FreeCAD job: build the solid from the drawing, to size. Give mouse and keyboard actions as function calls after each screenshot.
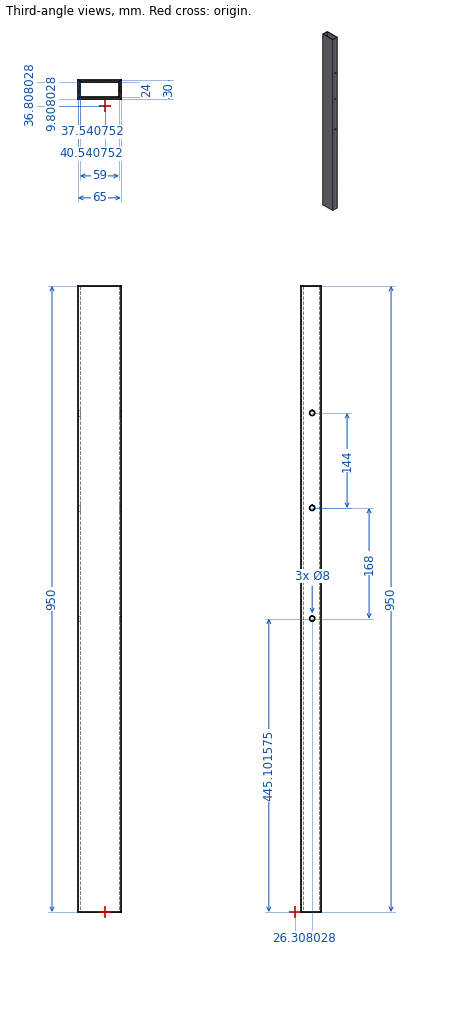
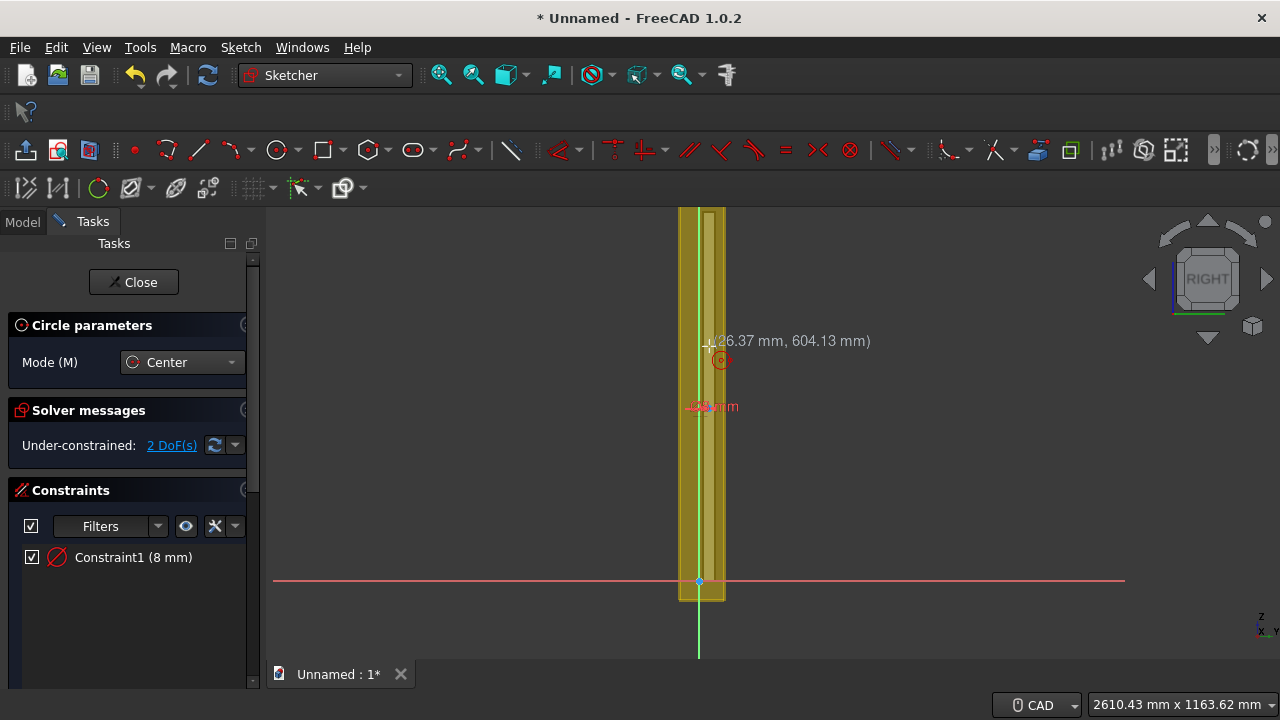
scroll(709, 343, up, 3)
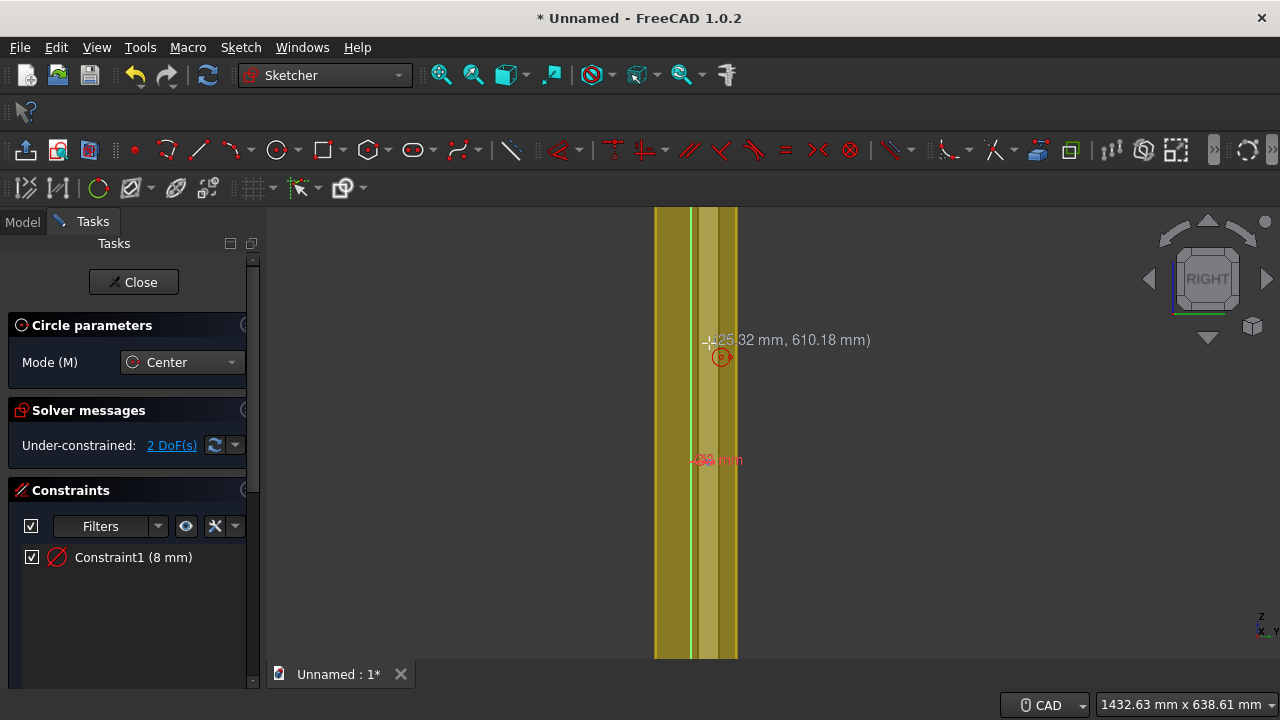
click(709, 343)
move(711, 341)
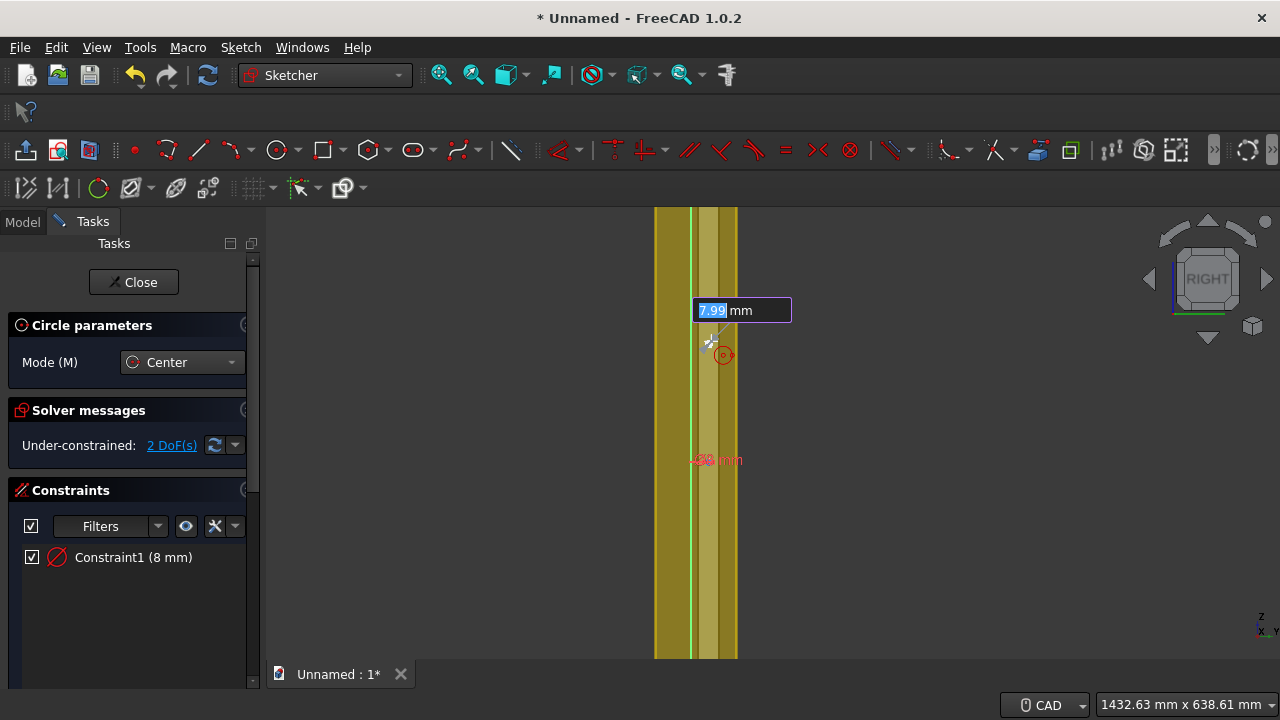
text(8)
key(Return)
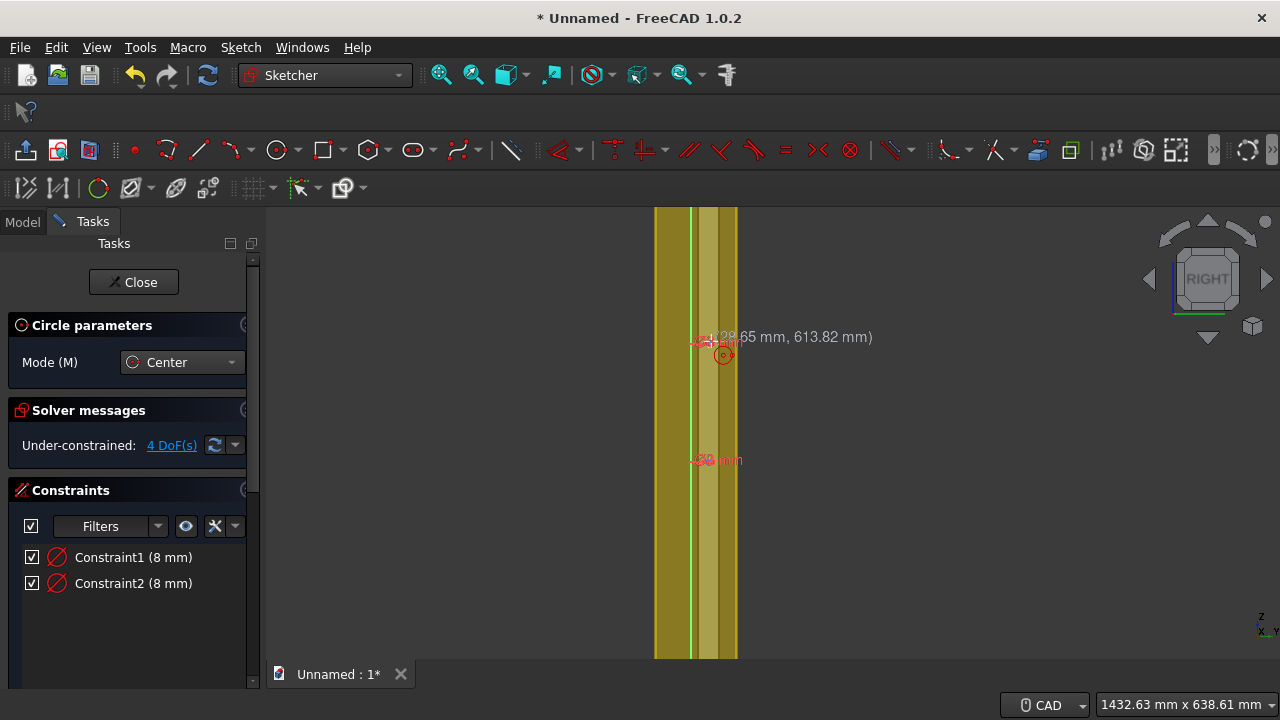
scroll(709, 241, up, 11)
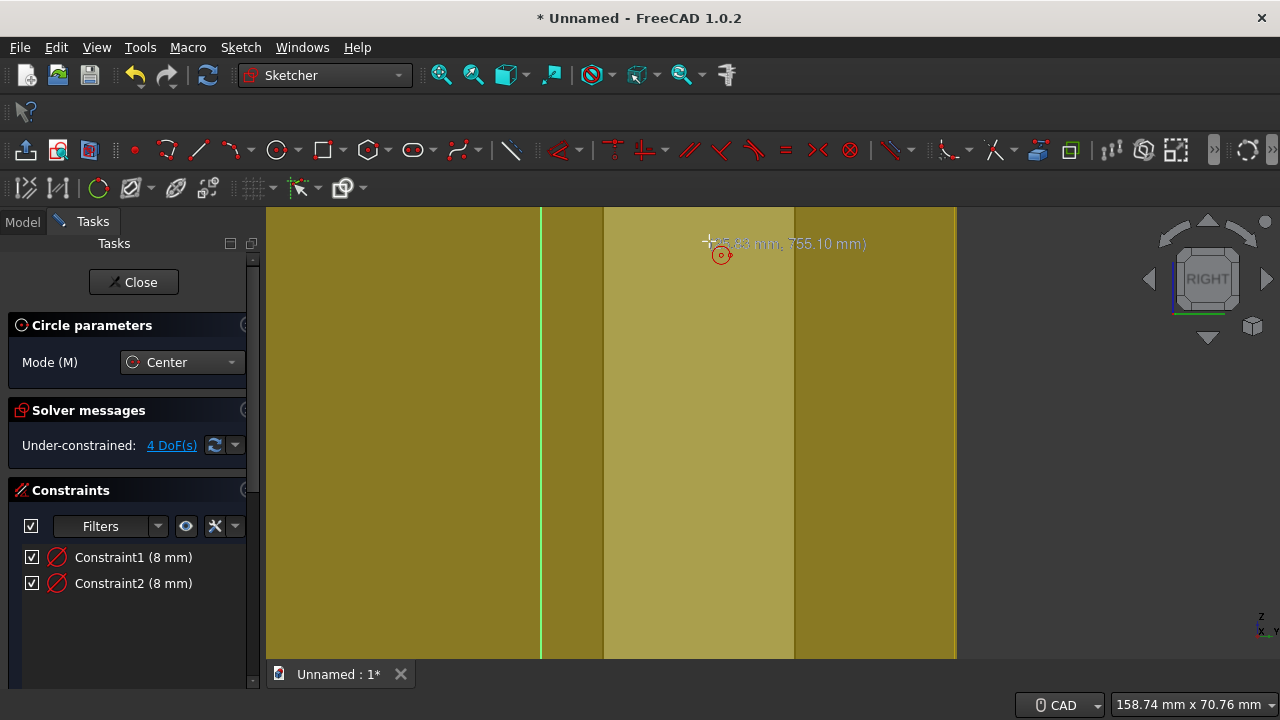
scroll(709, 290, down, 14)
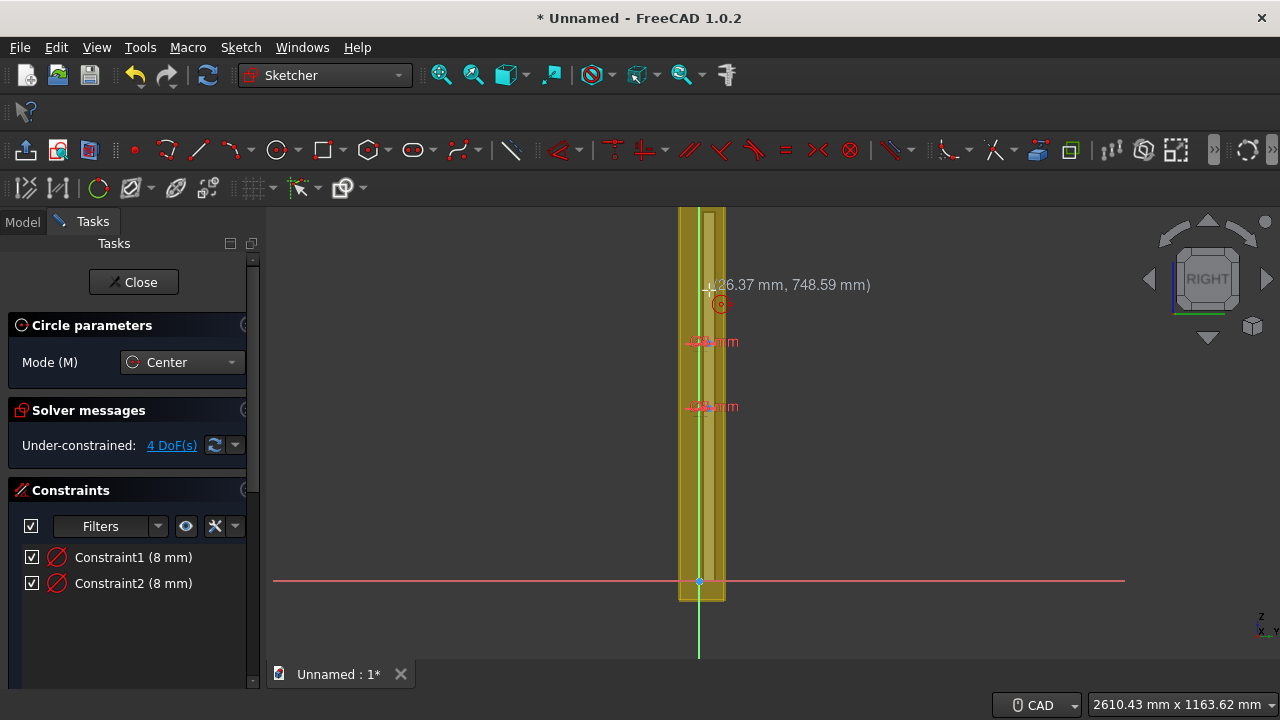
scroll(709, 287, up, 3)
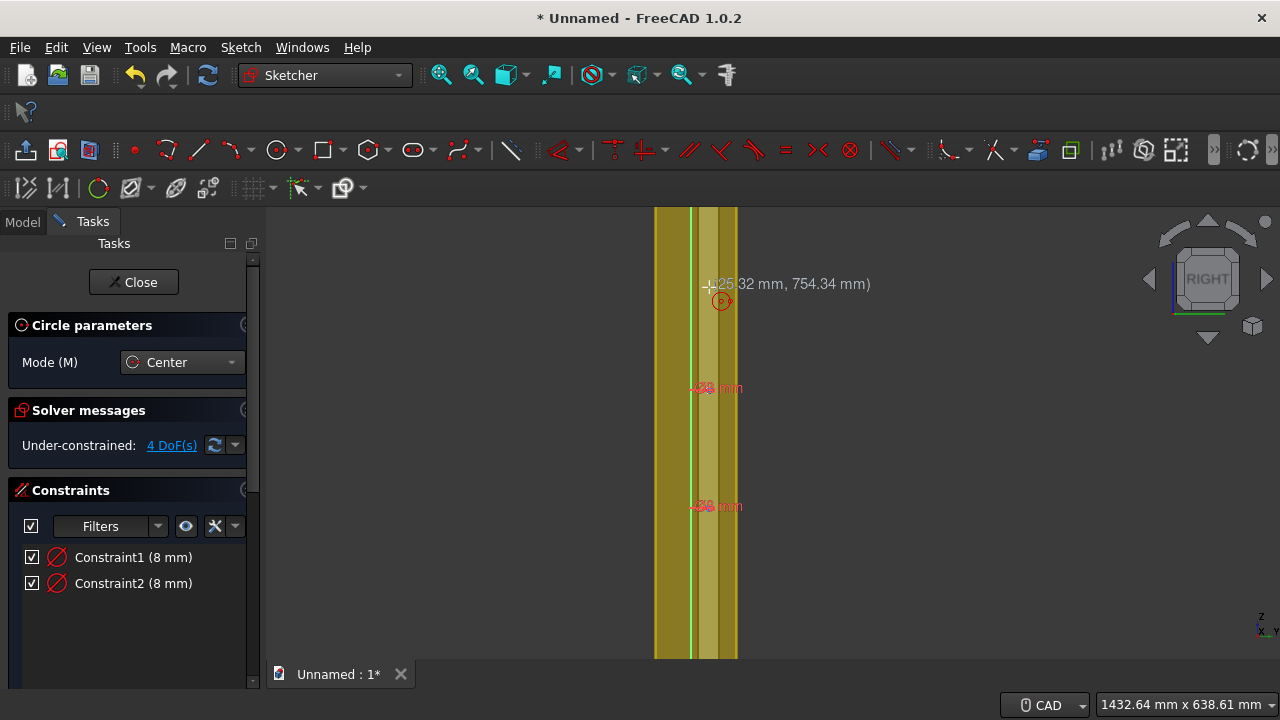
click(709, 287)
move(711, 285)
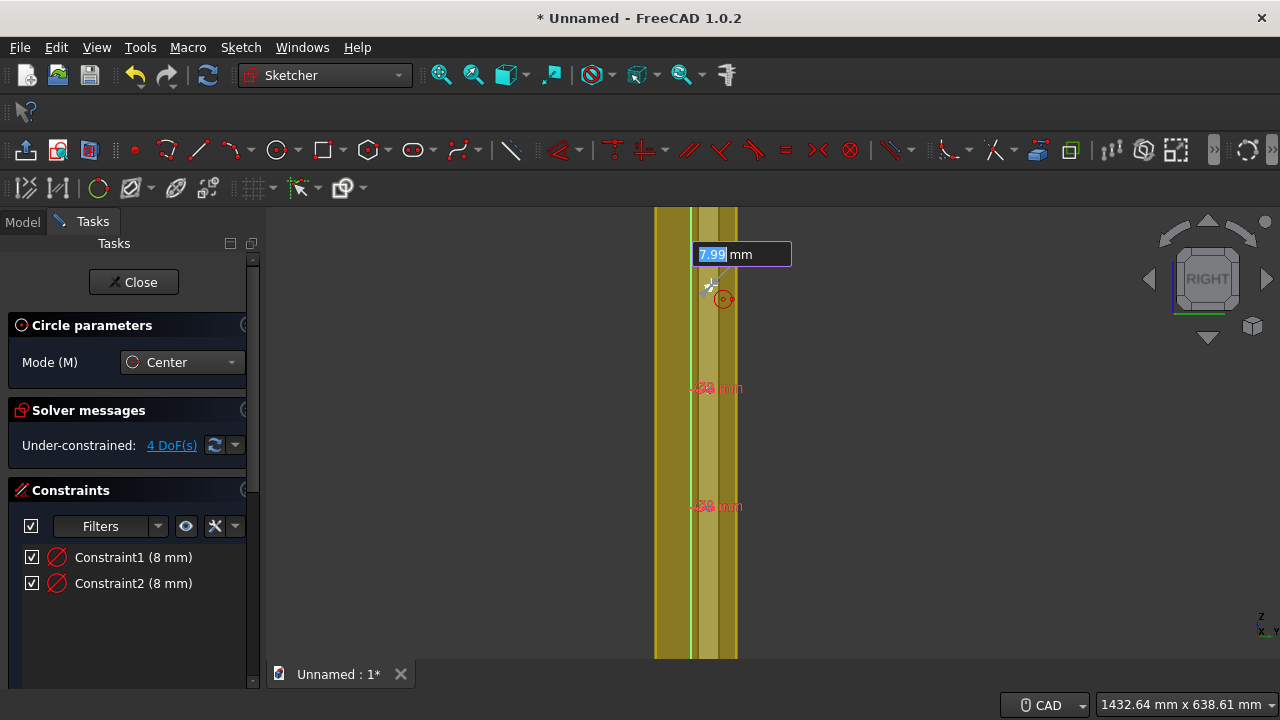
text(8)
key(Return)
key(Escape)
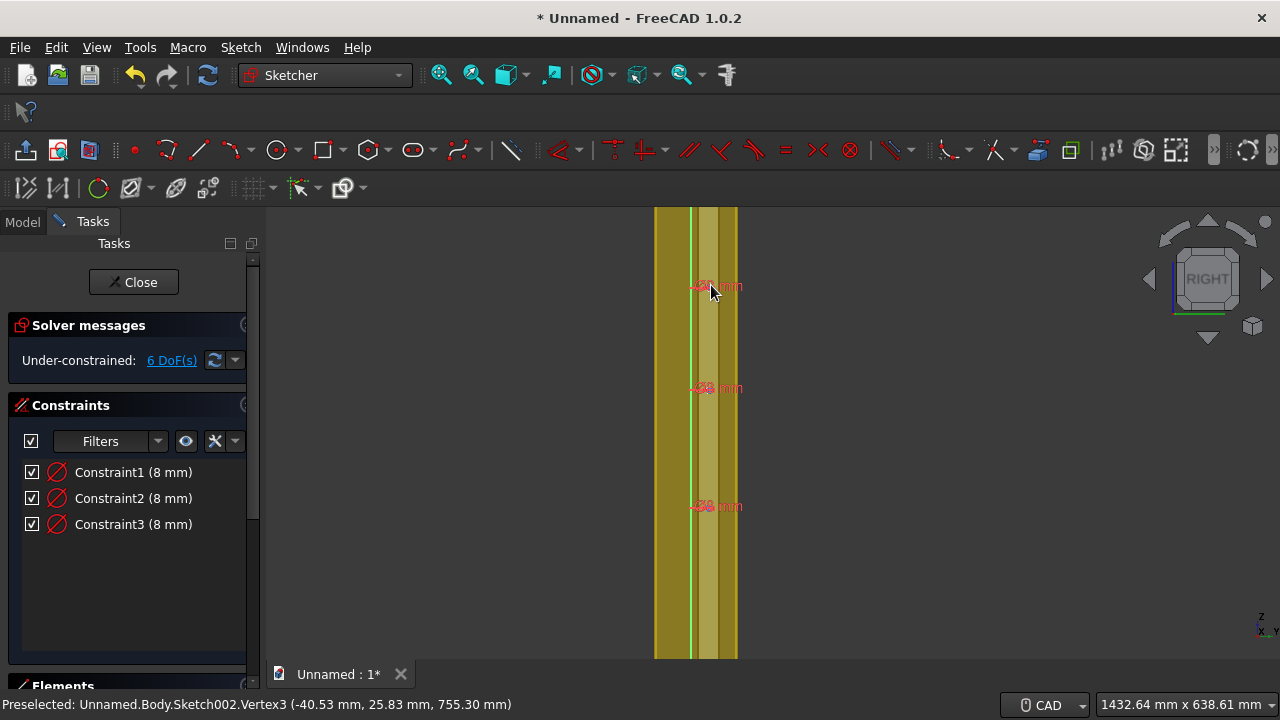
click(558, 150)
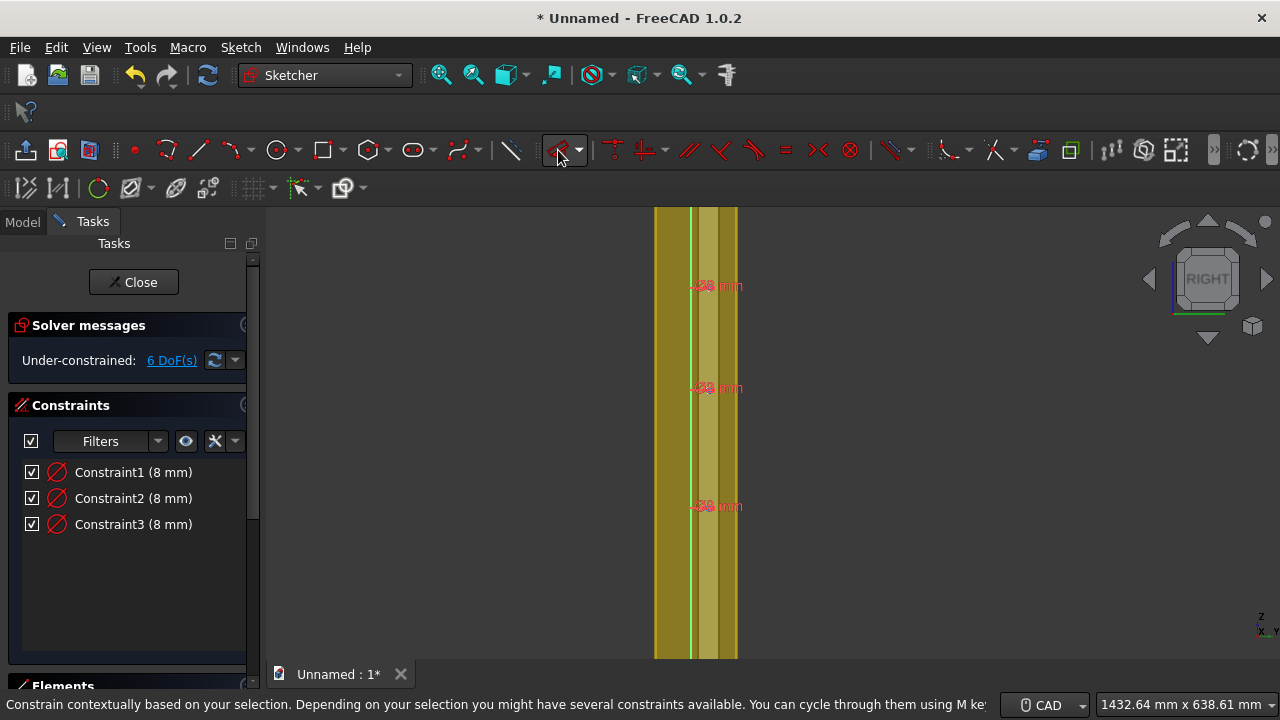
click(709, 508)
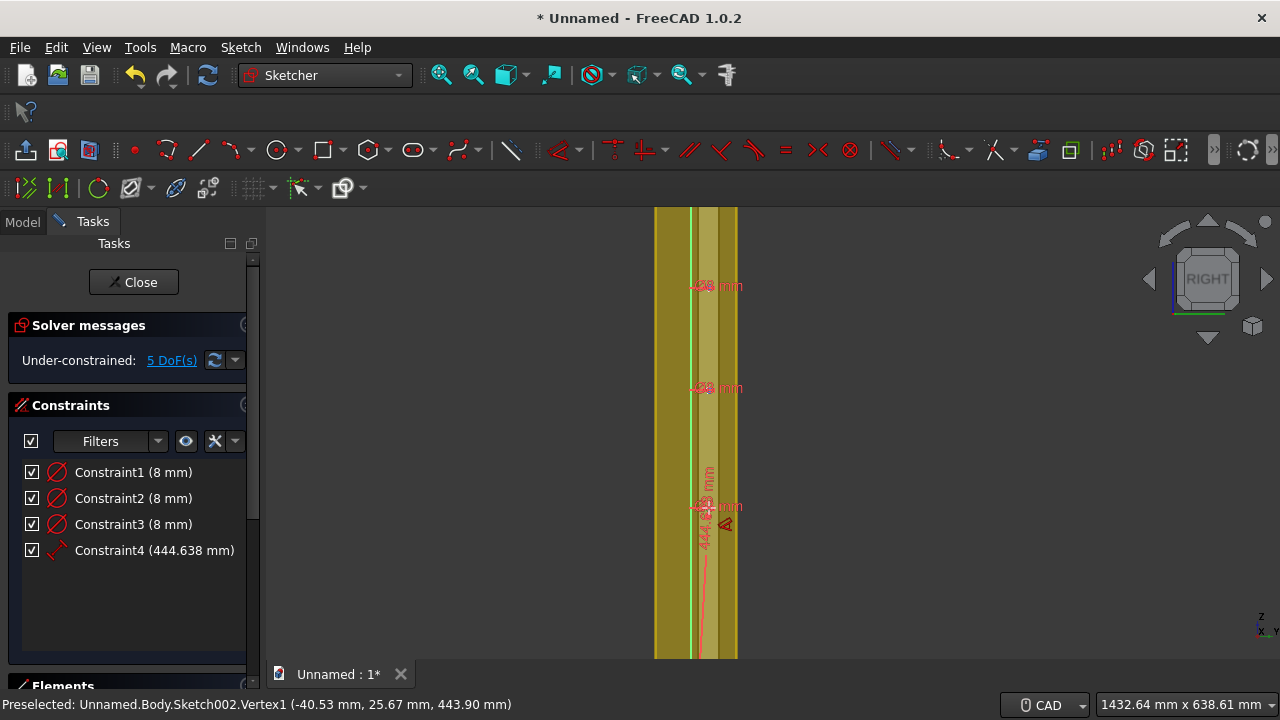
click(709, 390)
click(743, 449)